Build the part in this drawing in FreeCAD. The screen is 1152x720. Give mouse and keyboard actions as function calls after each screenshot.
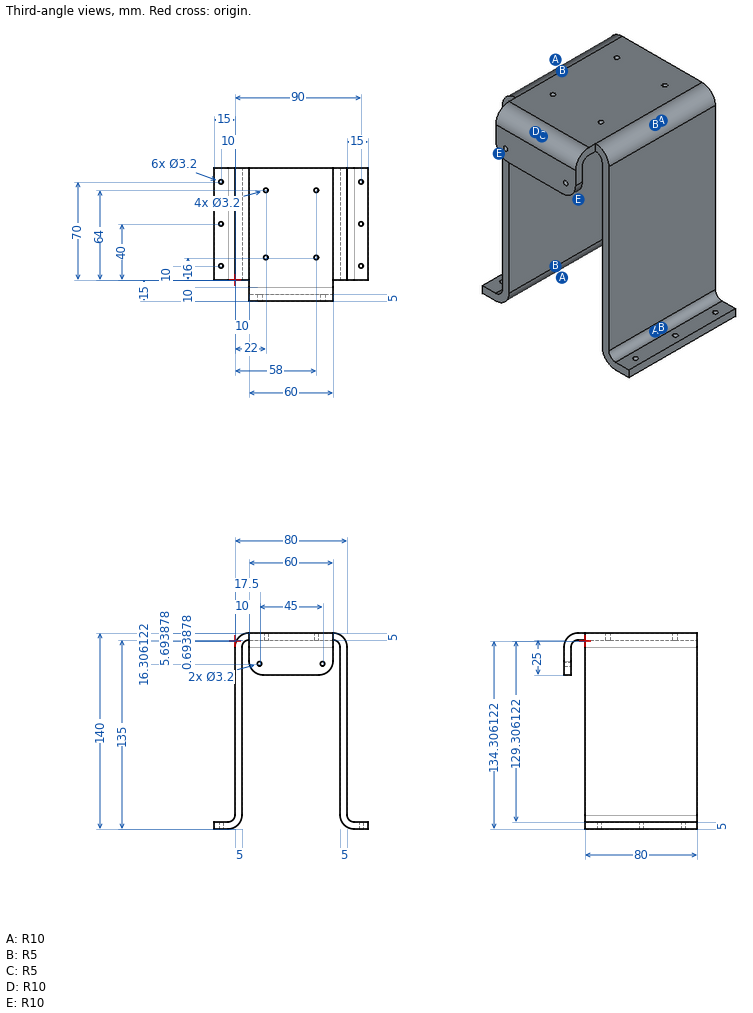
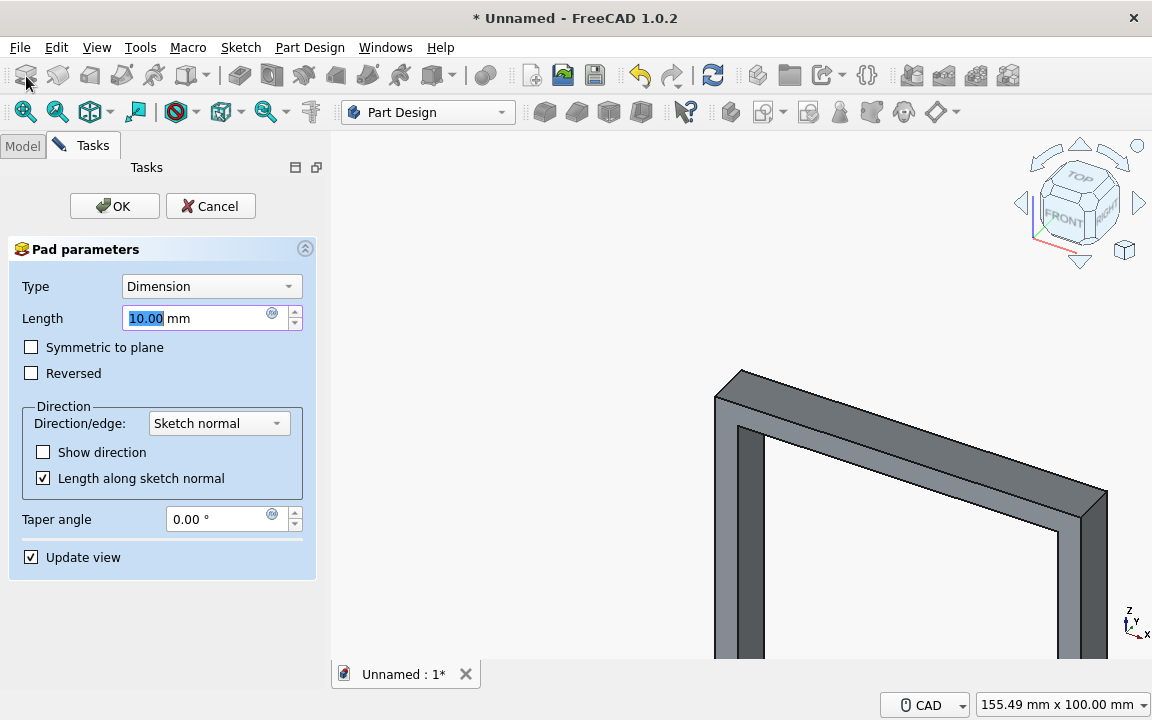
text(80)
key(Tab)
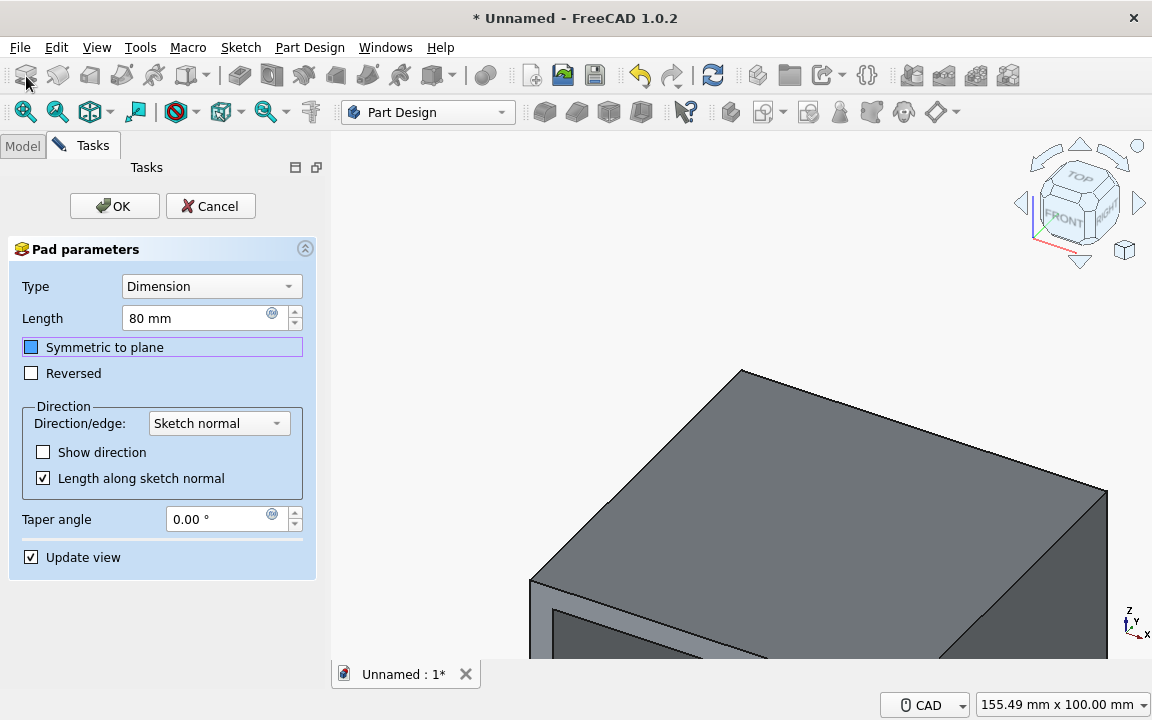
click(30, 373)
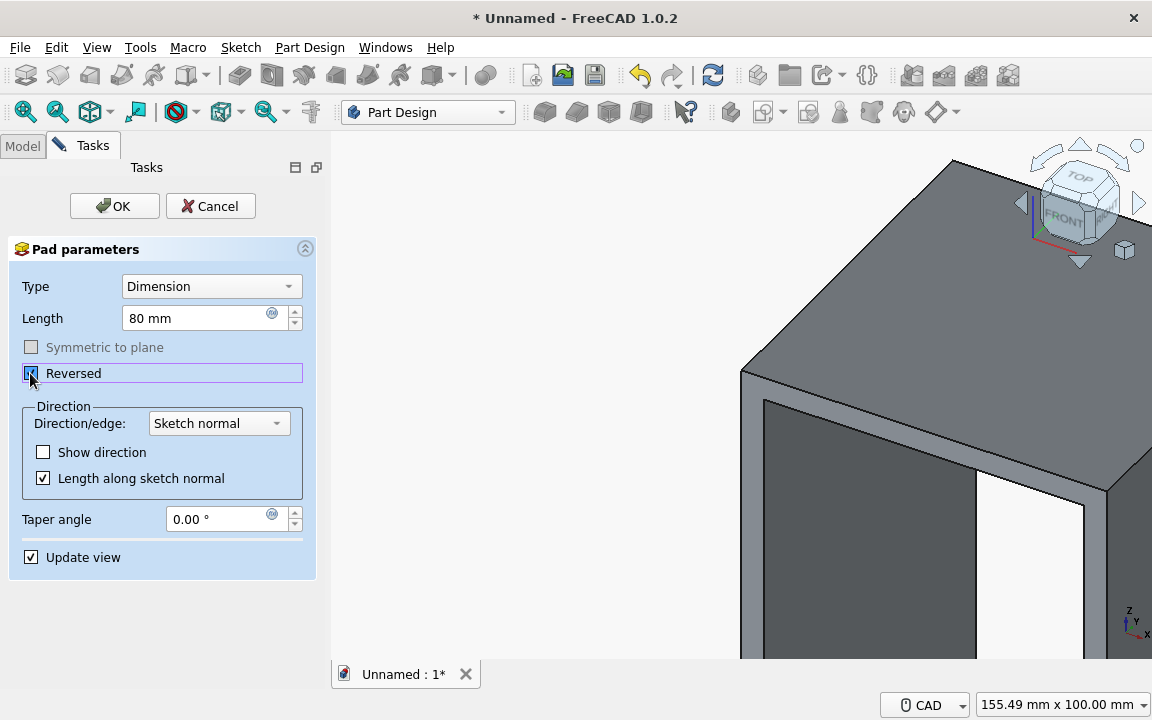
click(115, 206)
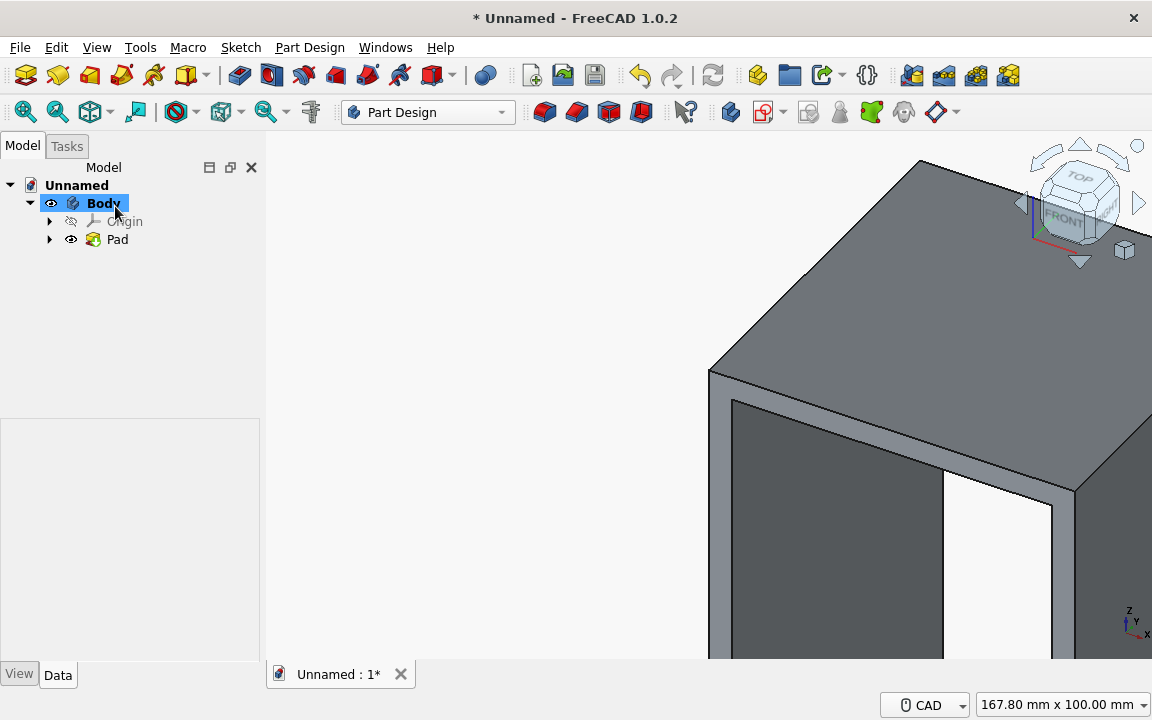
click(26, 112)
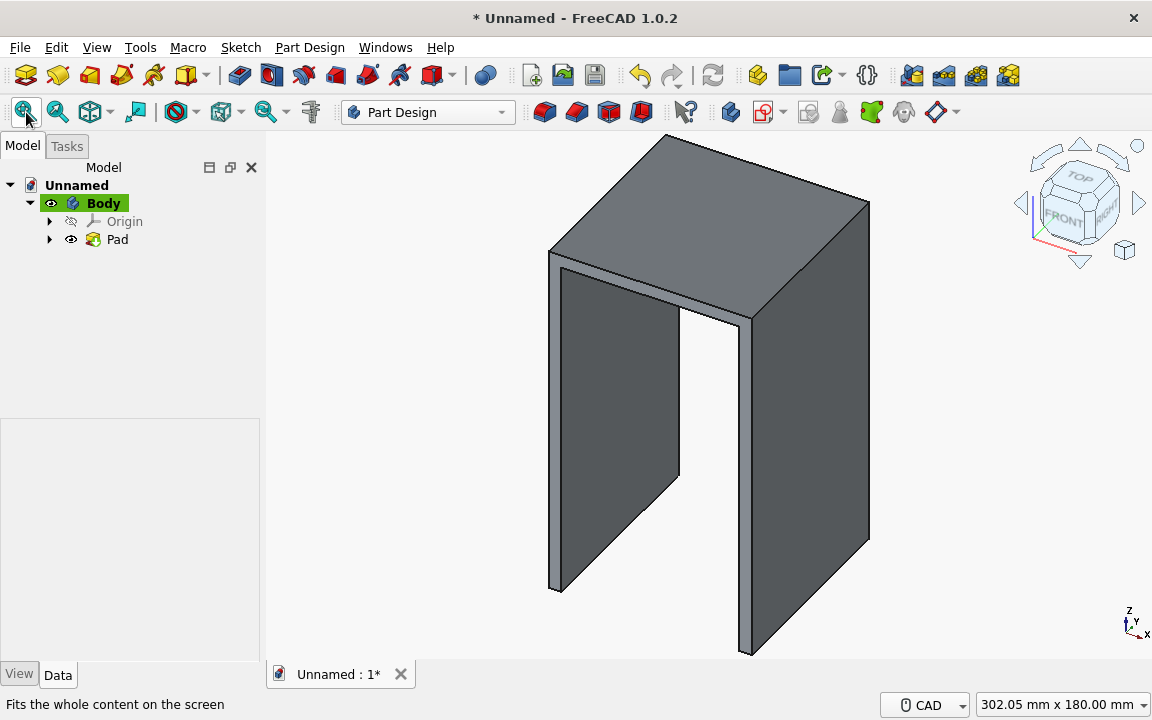
click(811, 428)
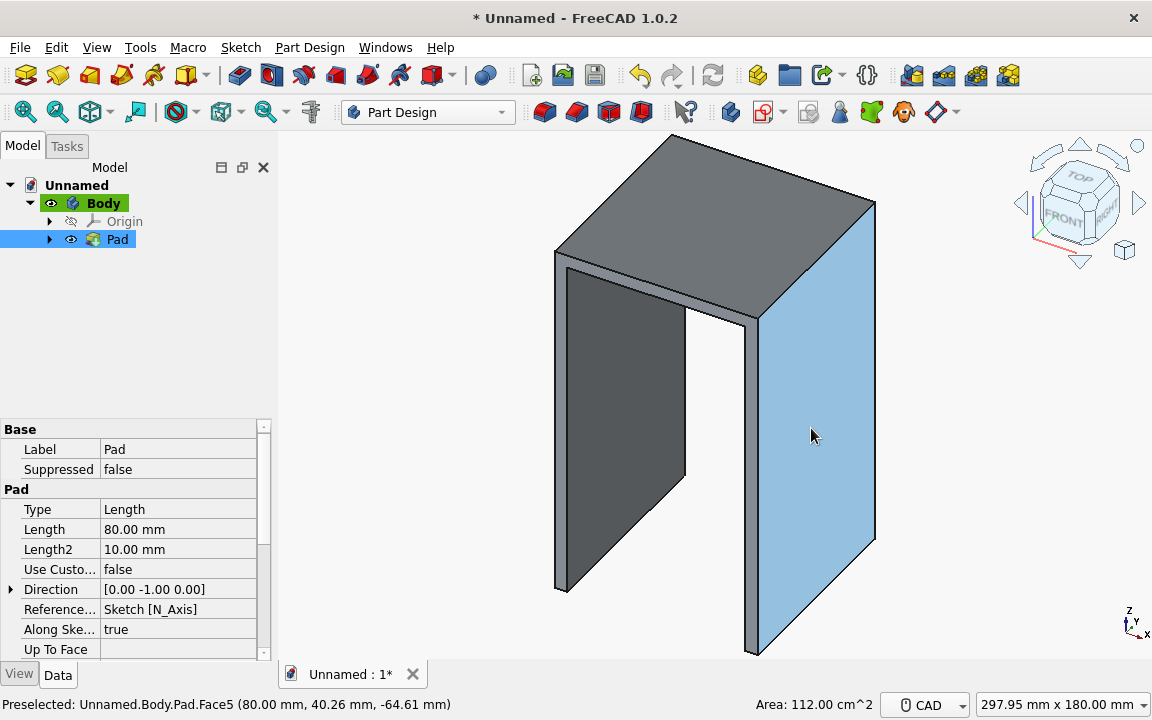
click(764, 112)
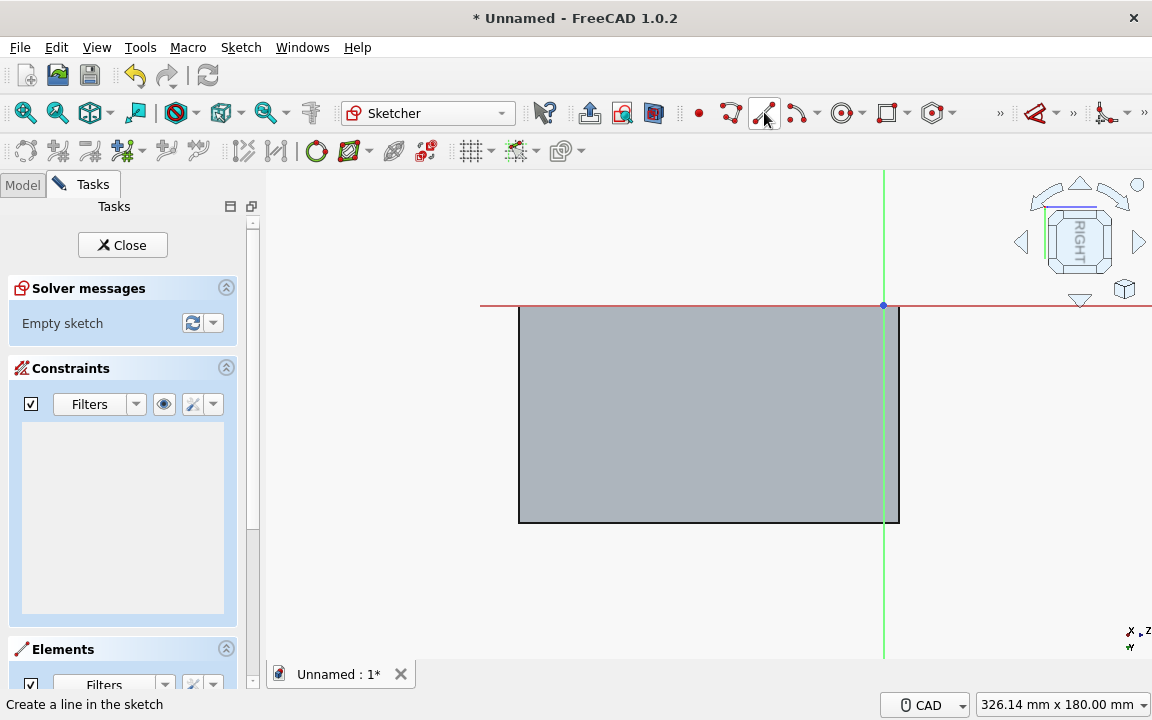
key(g)
key(r)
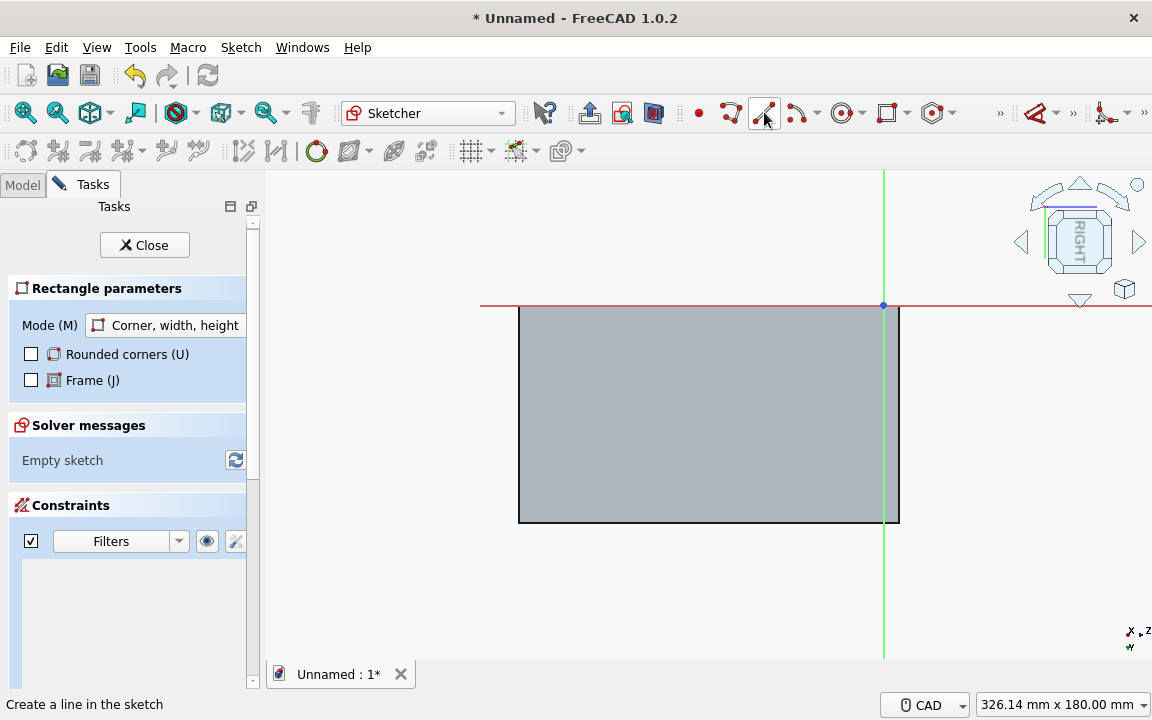
click(519, 306)
move(532, 523)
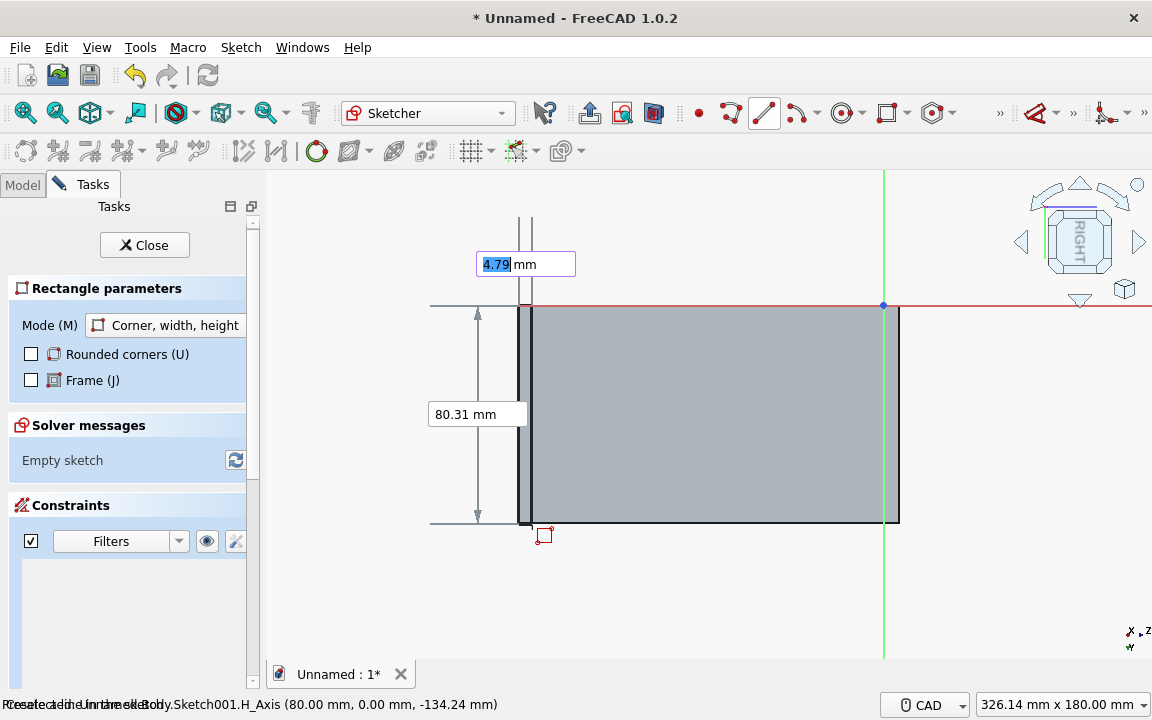
text(5)
key(Tab)
text(80)
key(Return)
key(Escape)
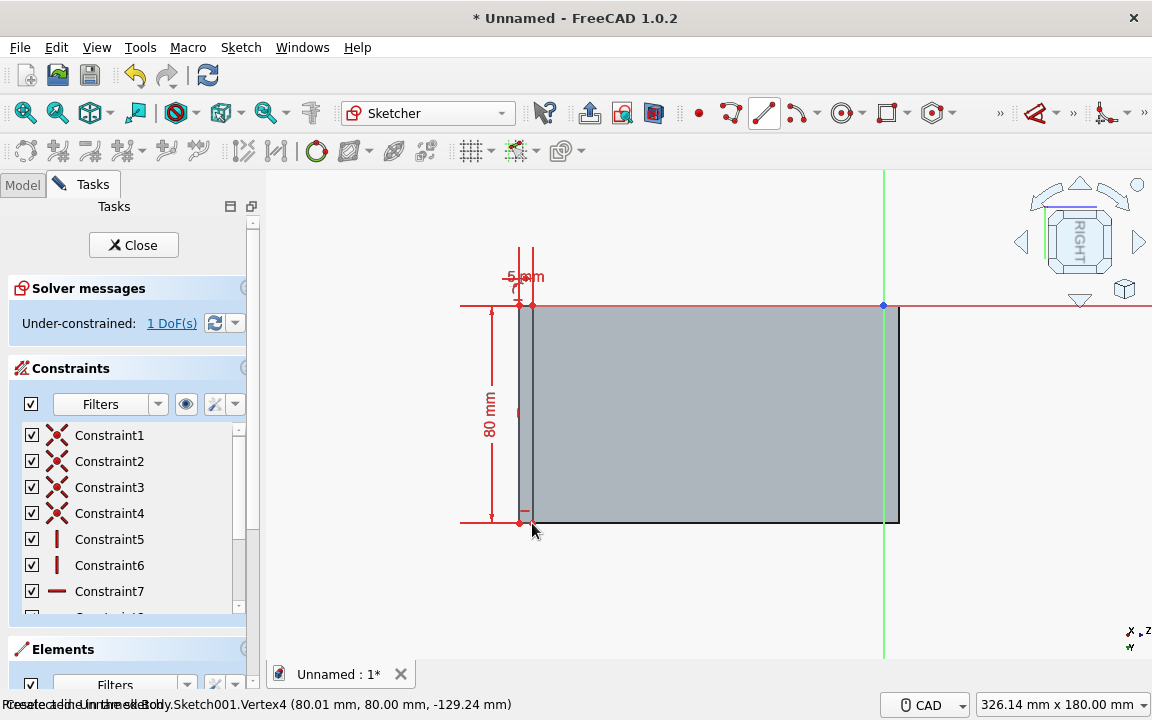
key(d)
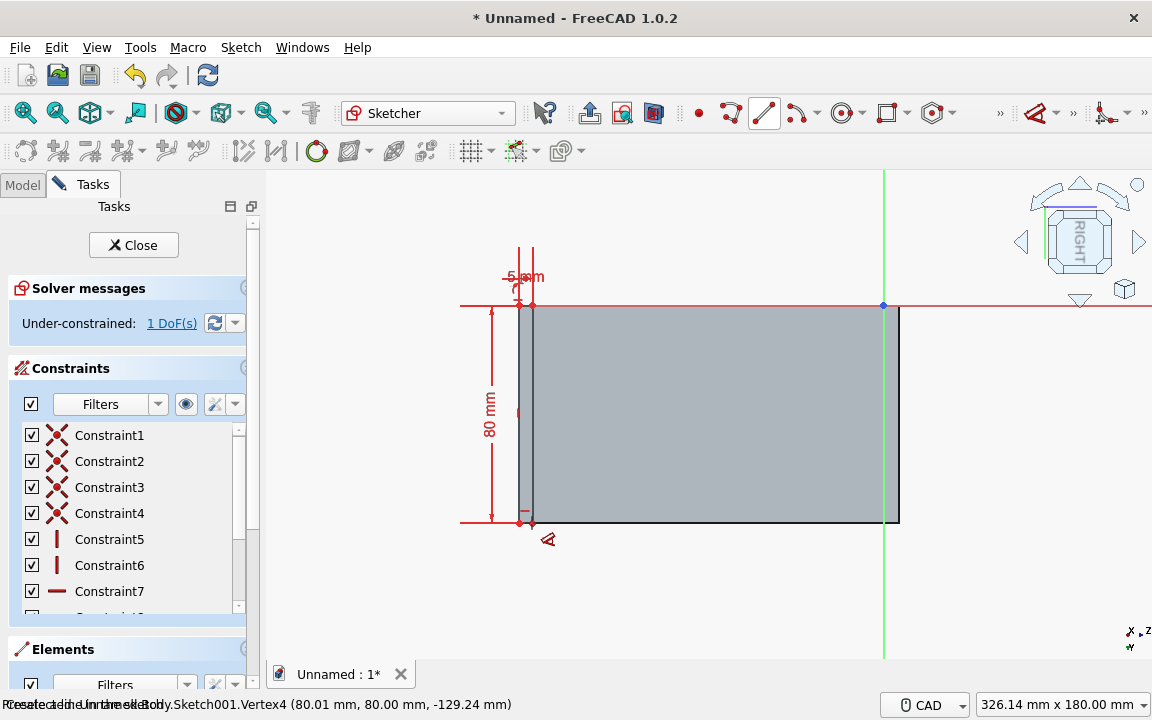
click(519, 306)
click(701, 272)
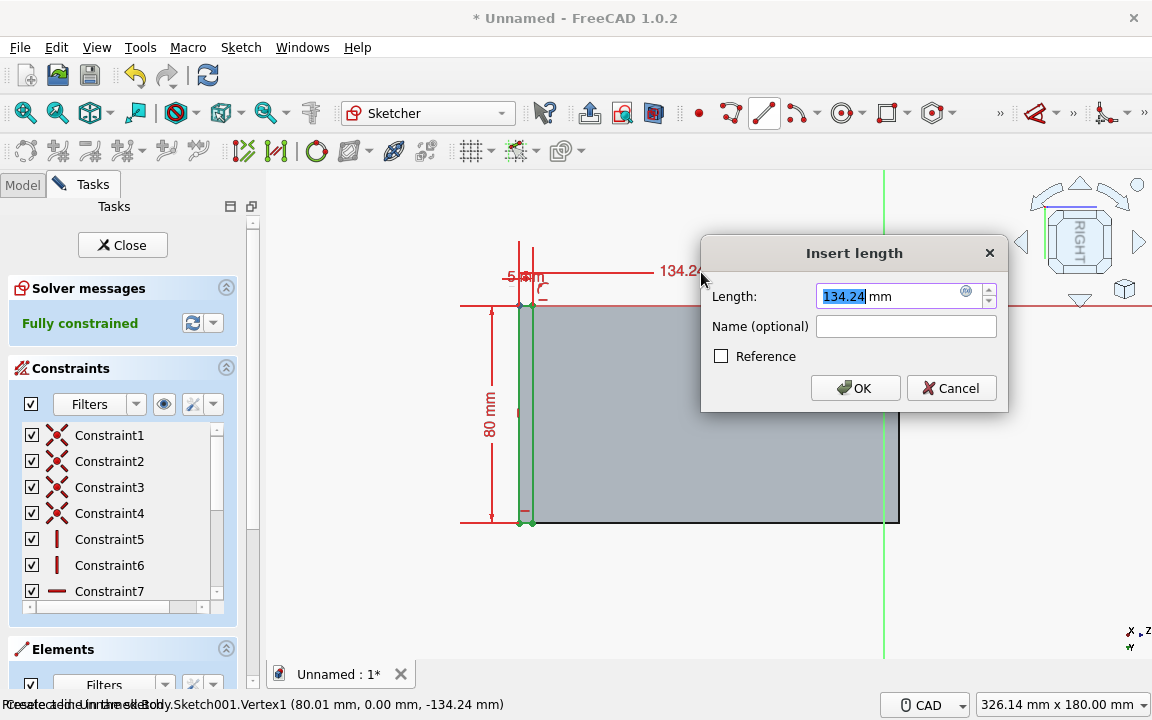
text(134.306122)
key(Return)
key(Escape)